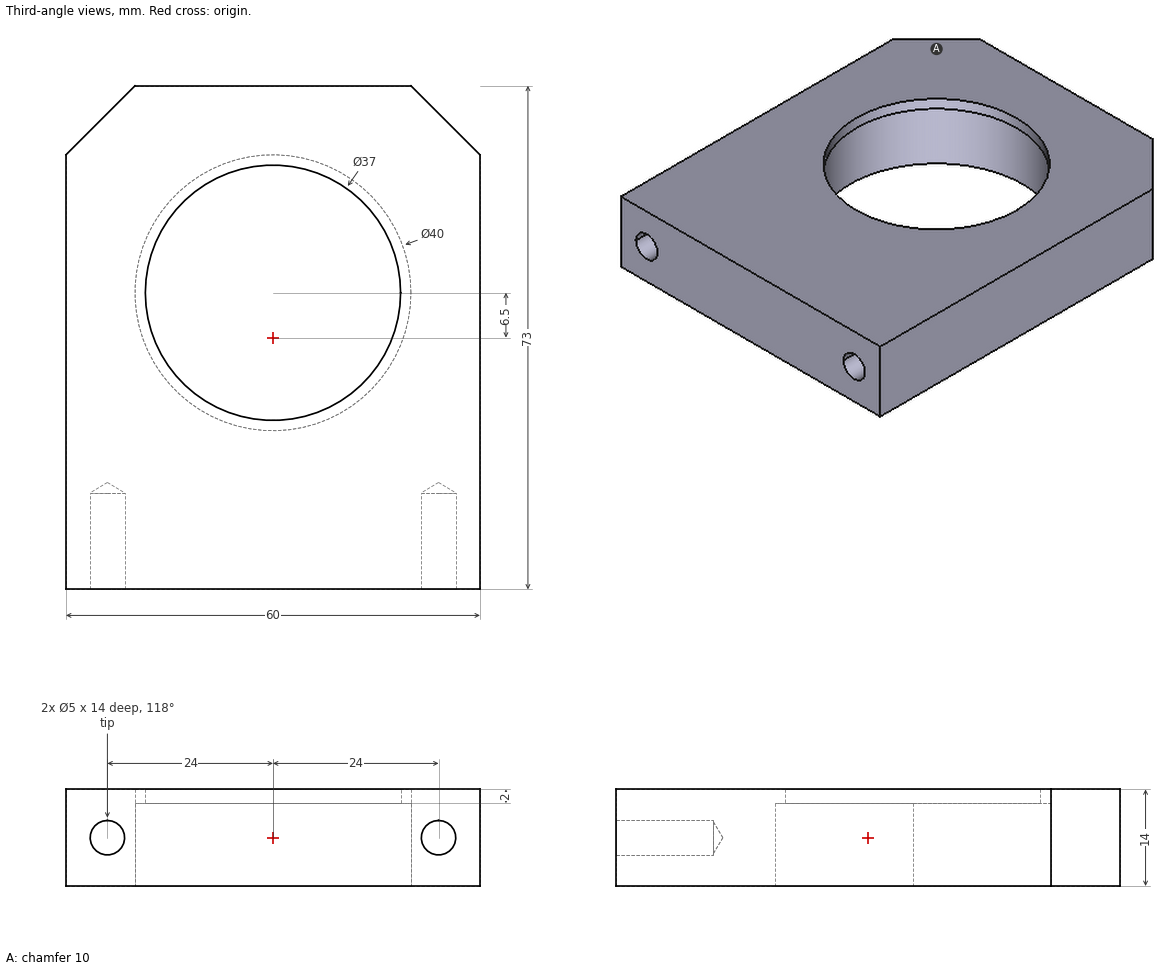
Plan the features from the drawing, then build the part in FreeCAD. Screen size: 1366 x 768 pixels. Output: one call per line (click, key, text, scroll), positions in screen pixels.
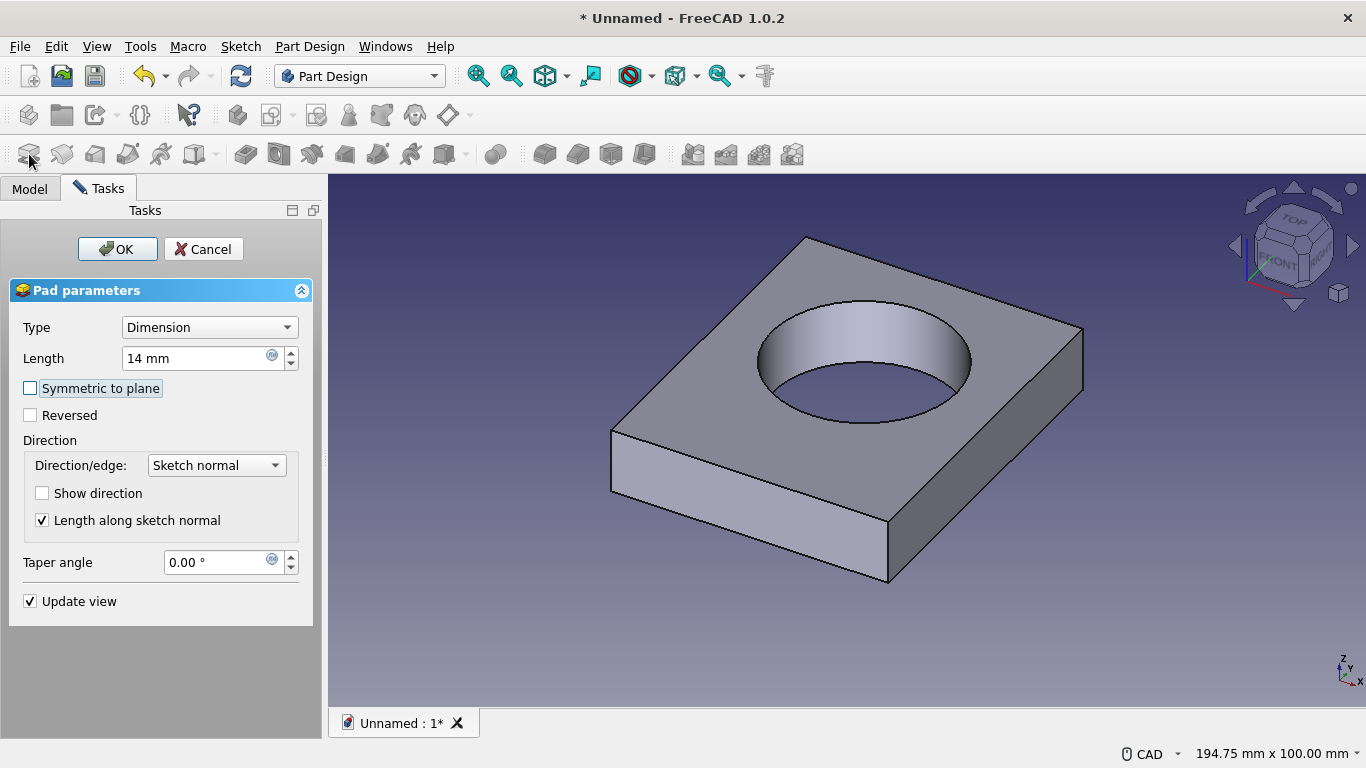
click(31, 388)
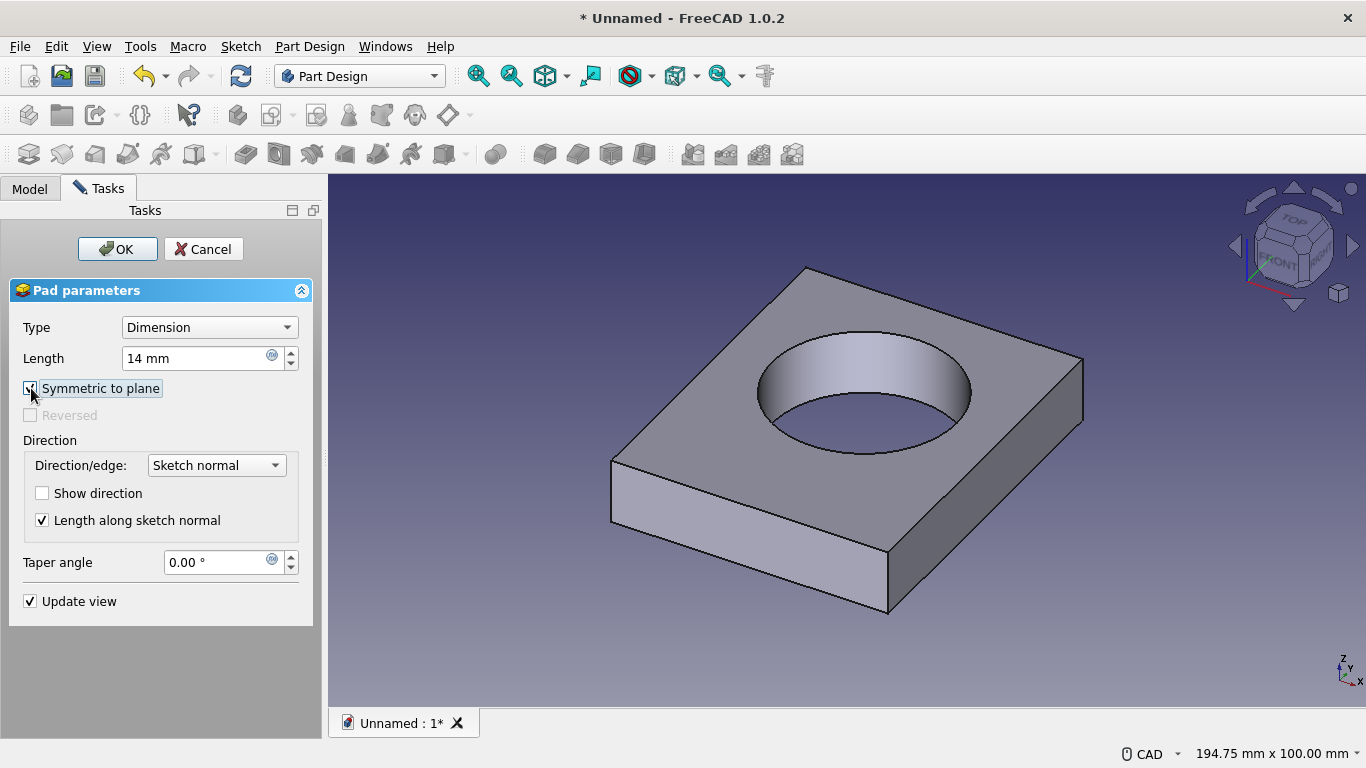
click(118, 249)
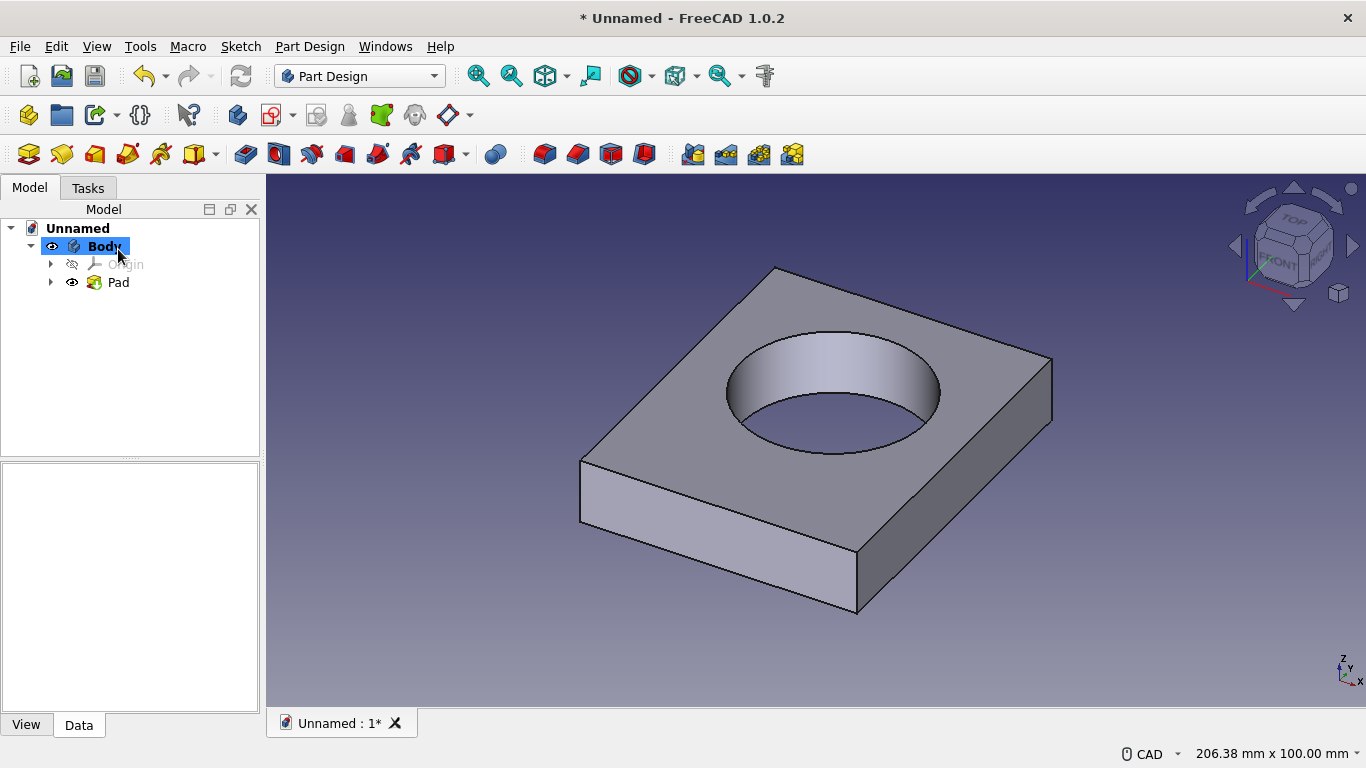
click(51, 264)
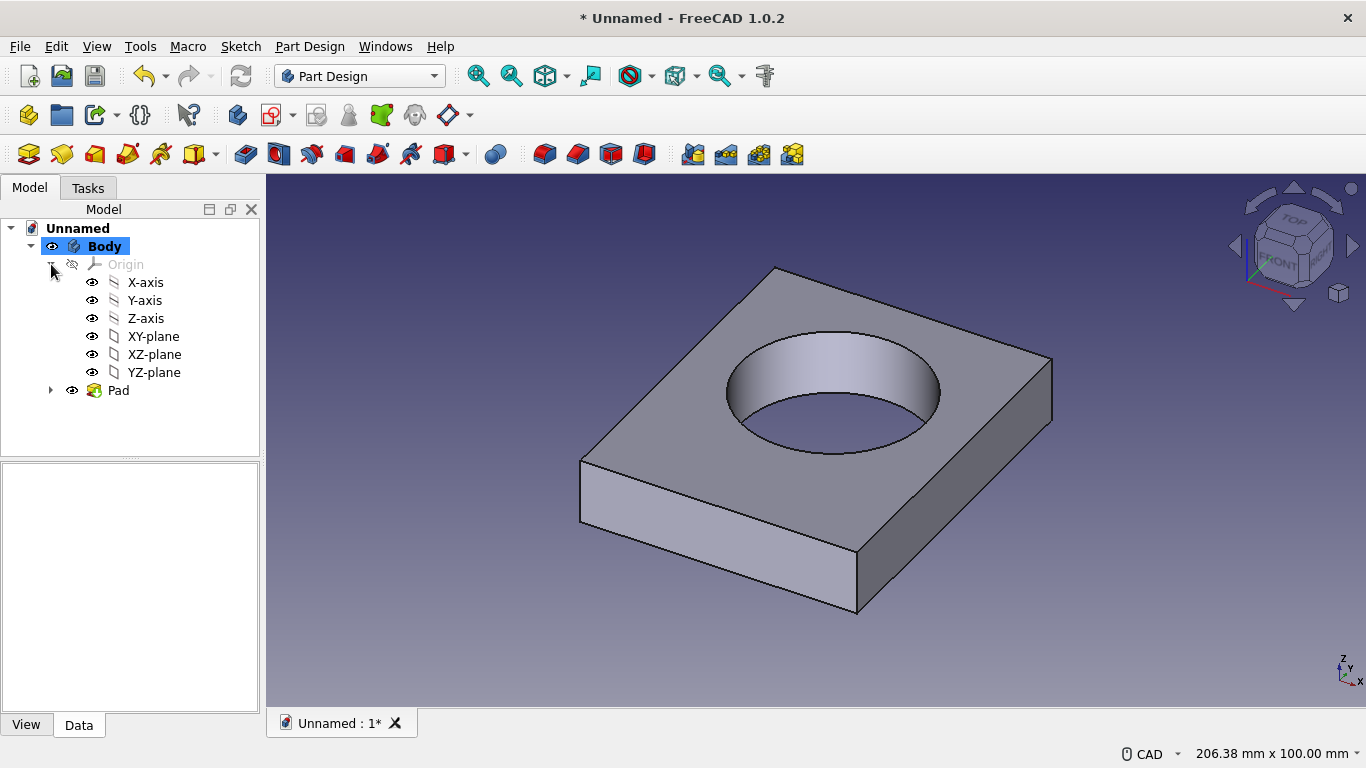
click(137, 336)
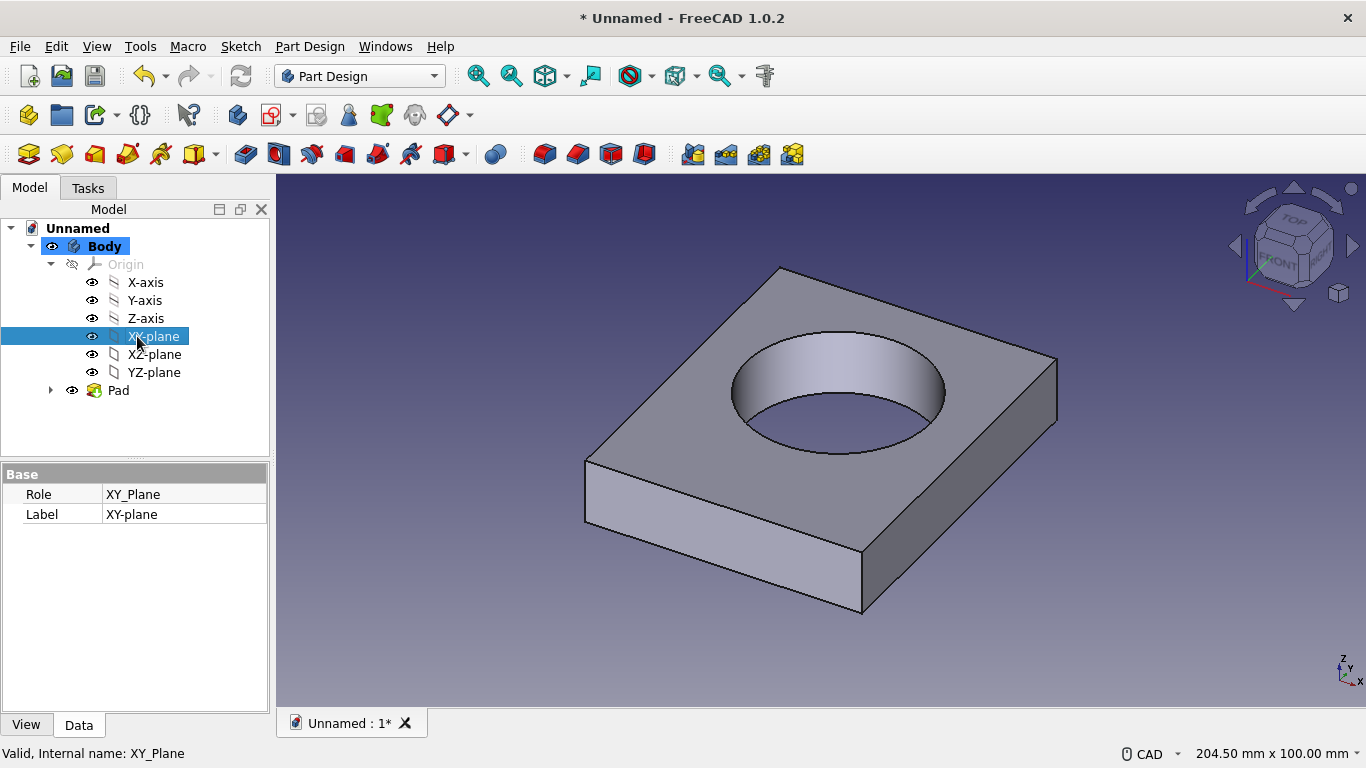
click(448, 116)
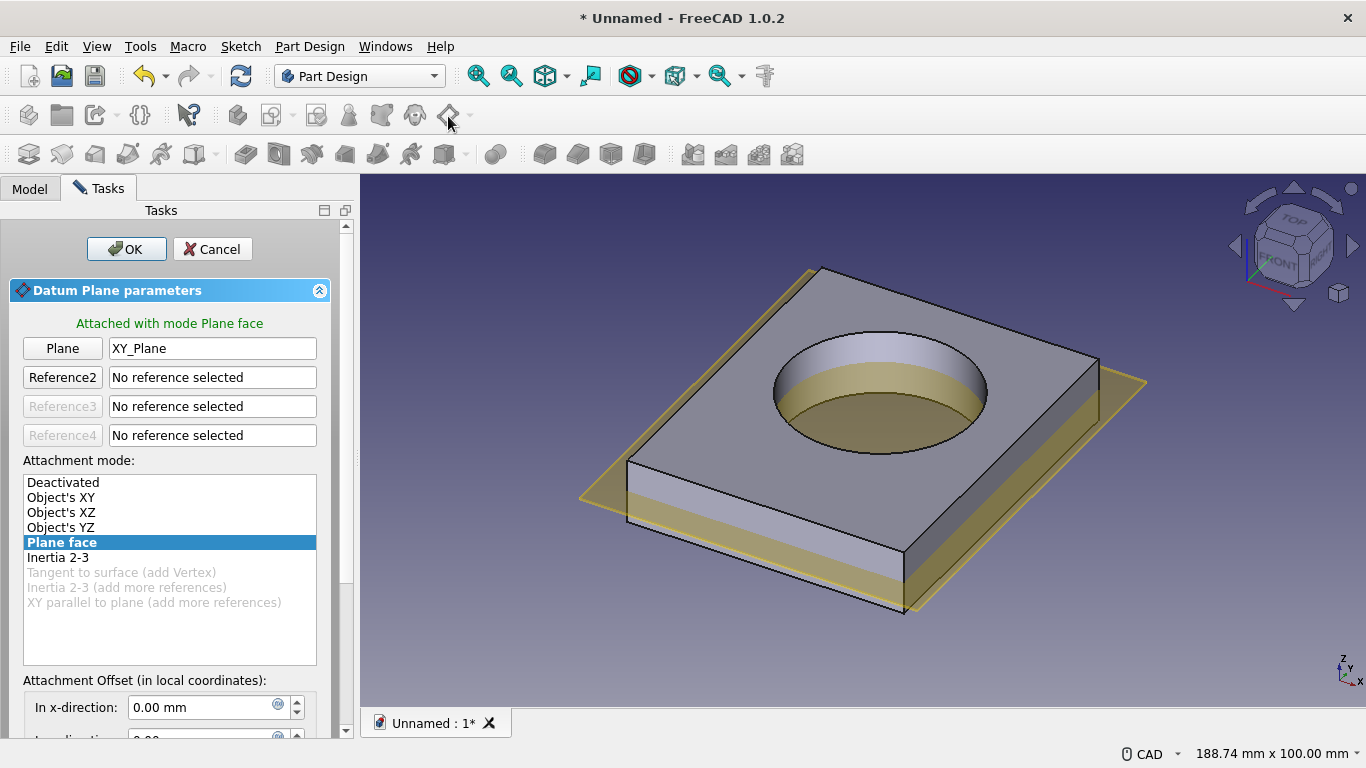
scroll(346, 479, down, 2)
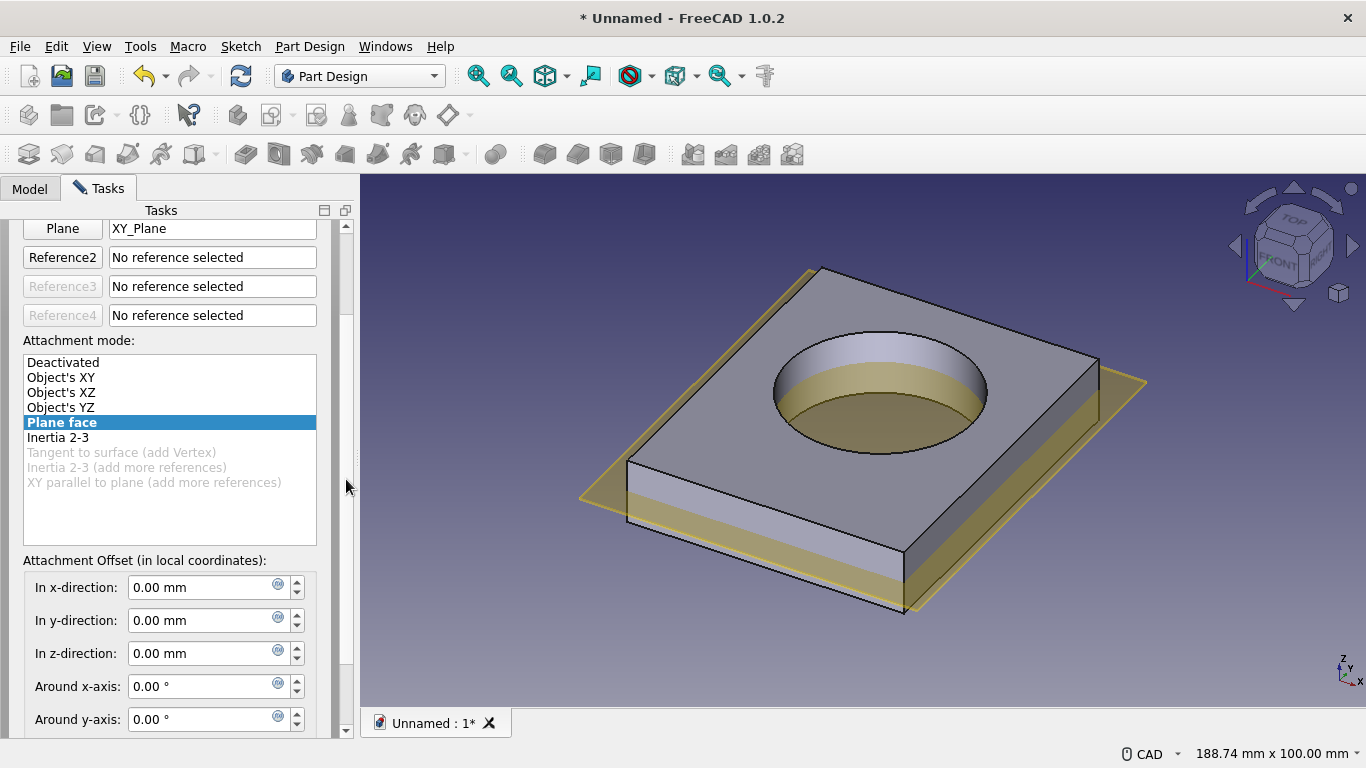
triple_click(210, 654)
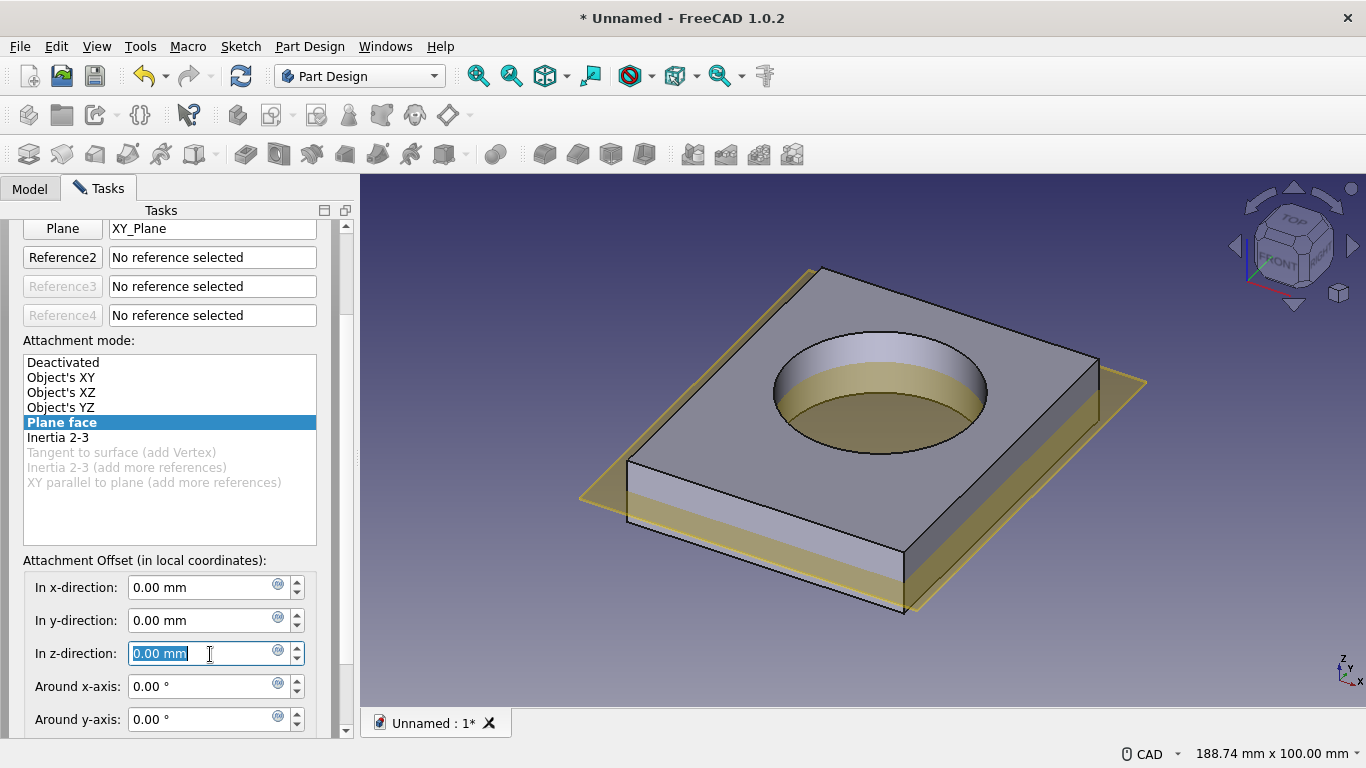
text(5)
key(Tab)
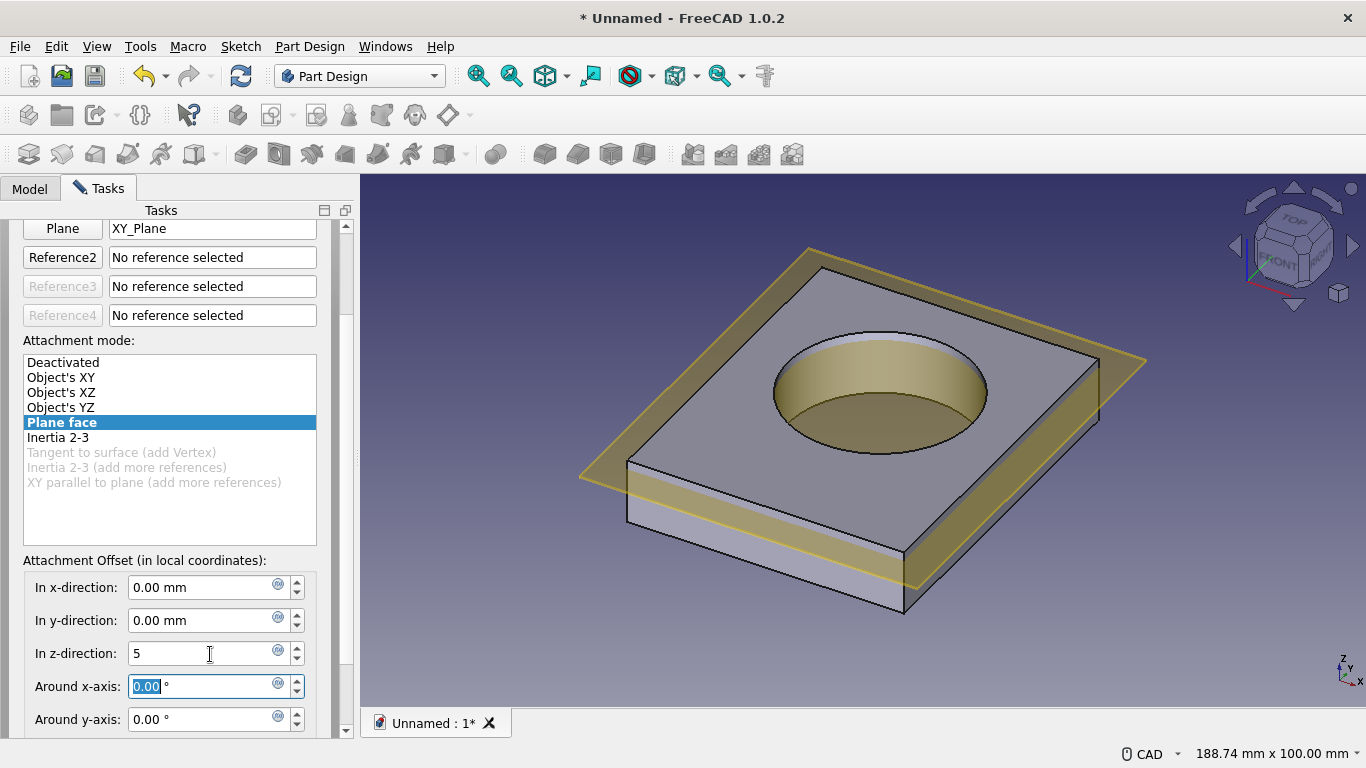
scroll(346, 479, up, 3)